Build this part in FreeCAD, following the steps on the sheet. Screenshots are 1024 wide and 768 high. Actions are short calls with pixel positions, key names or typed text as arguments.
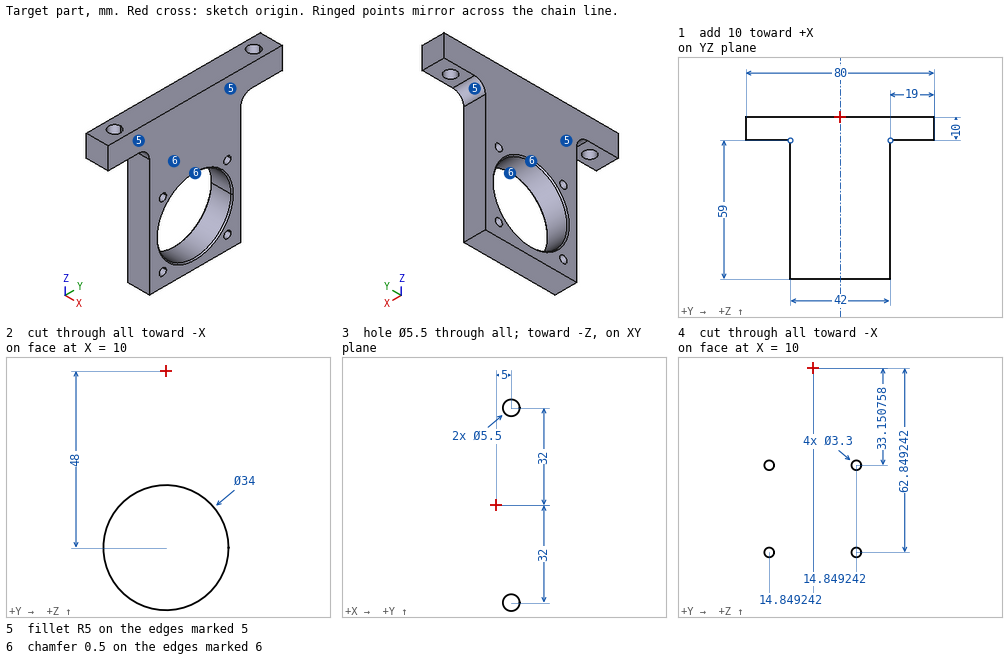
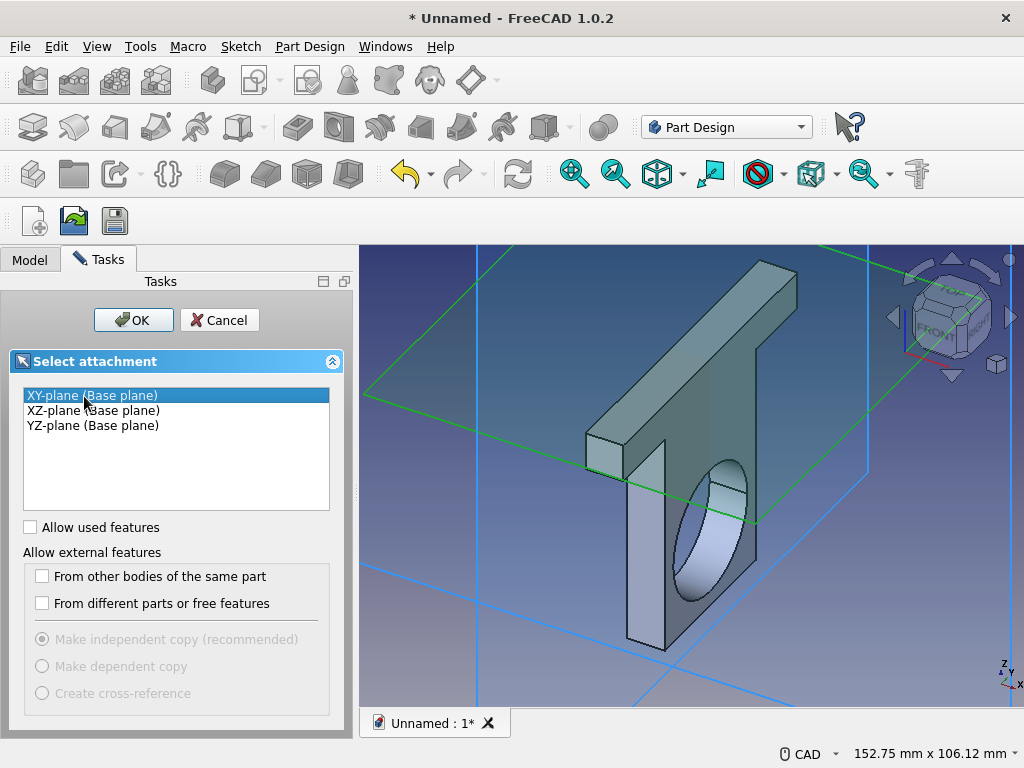
click(134, 320)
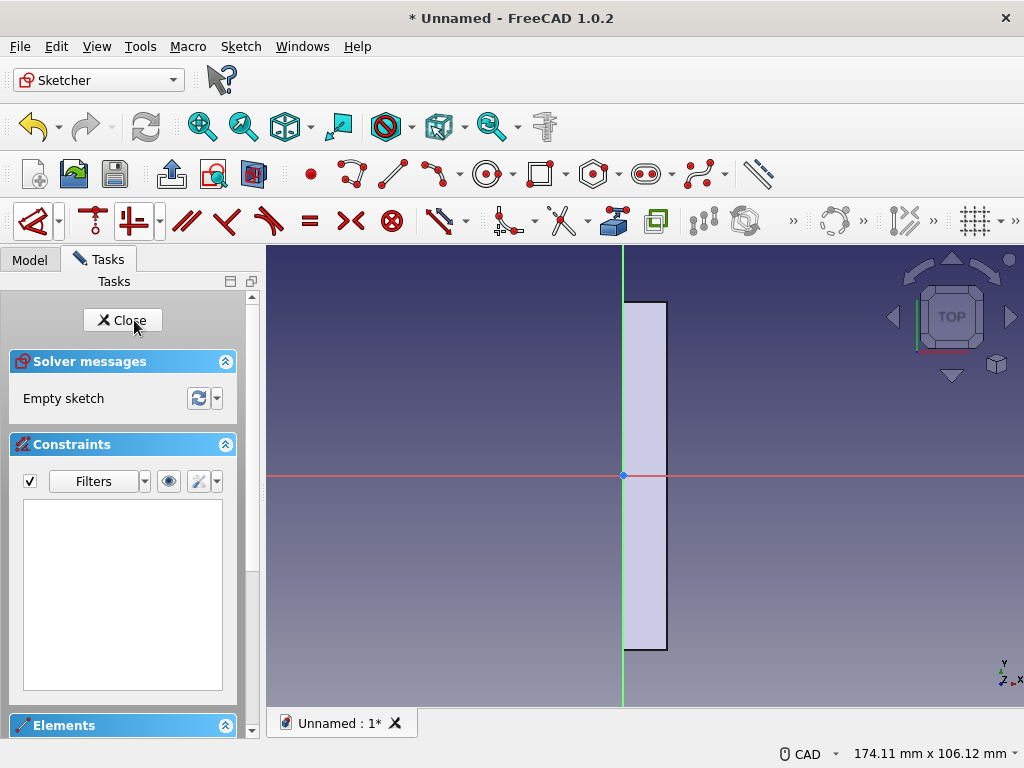
click(486, 174)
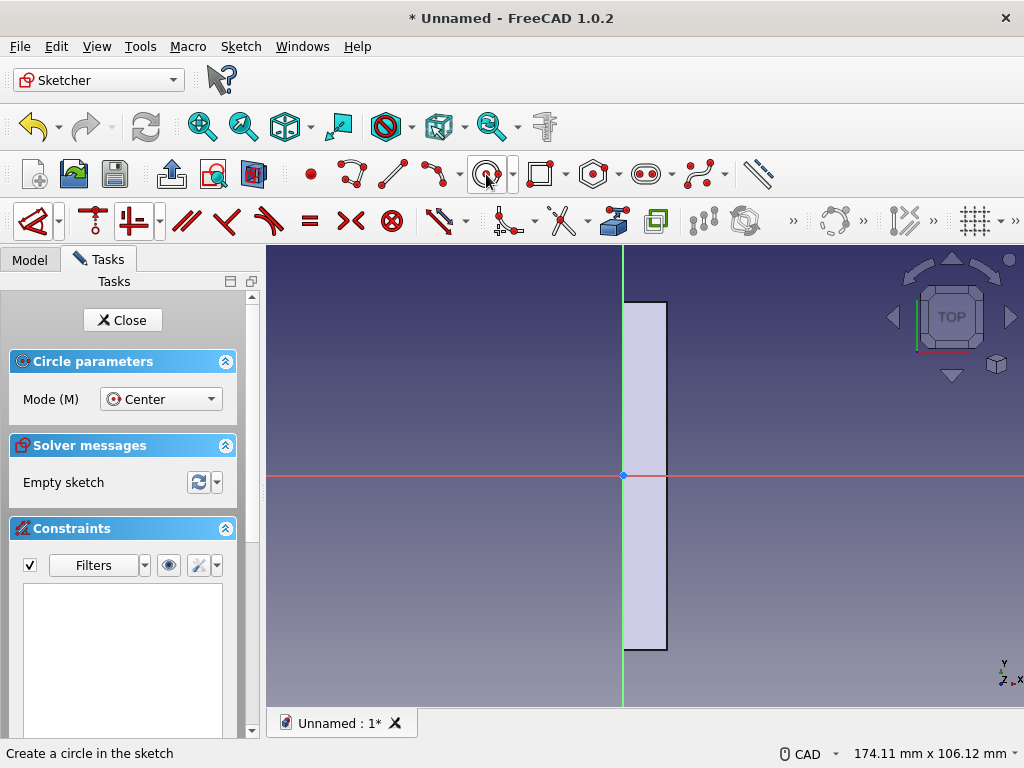
scroll(645, 337, up, 4)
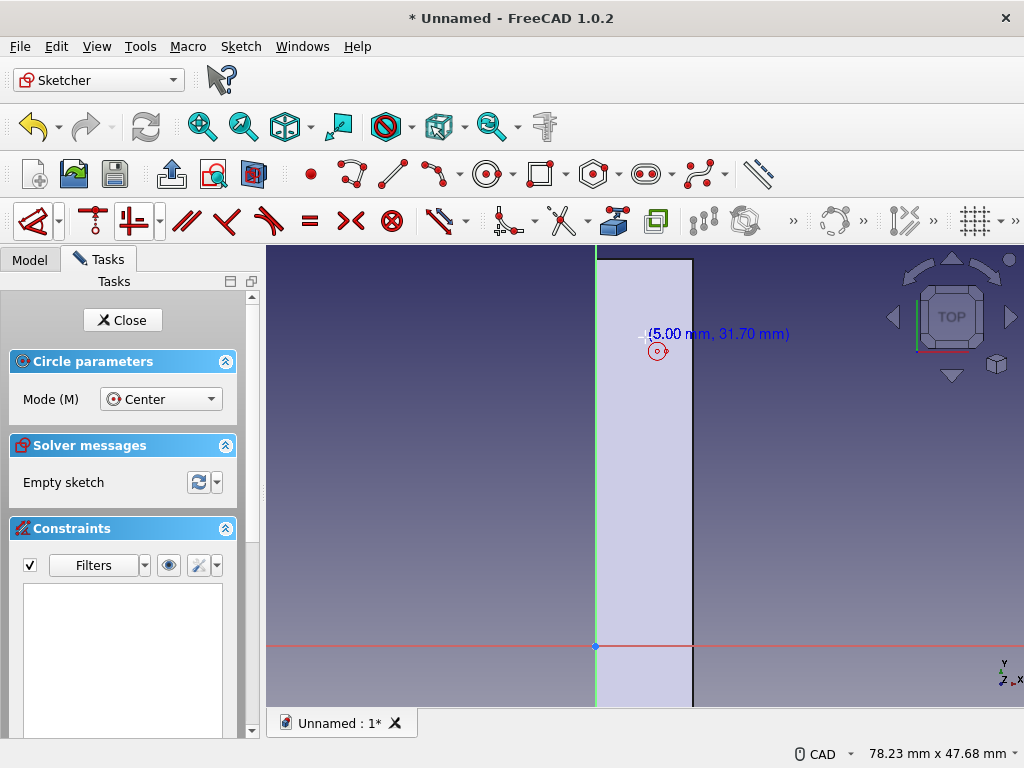
click(644, 336)
move(663, 317)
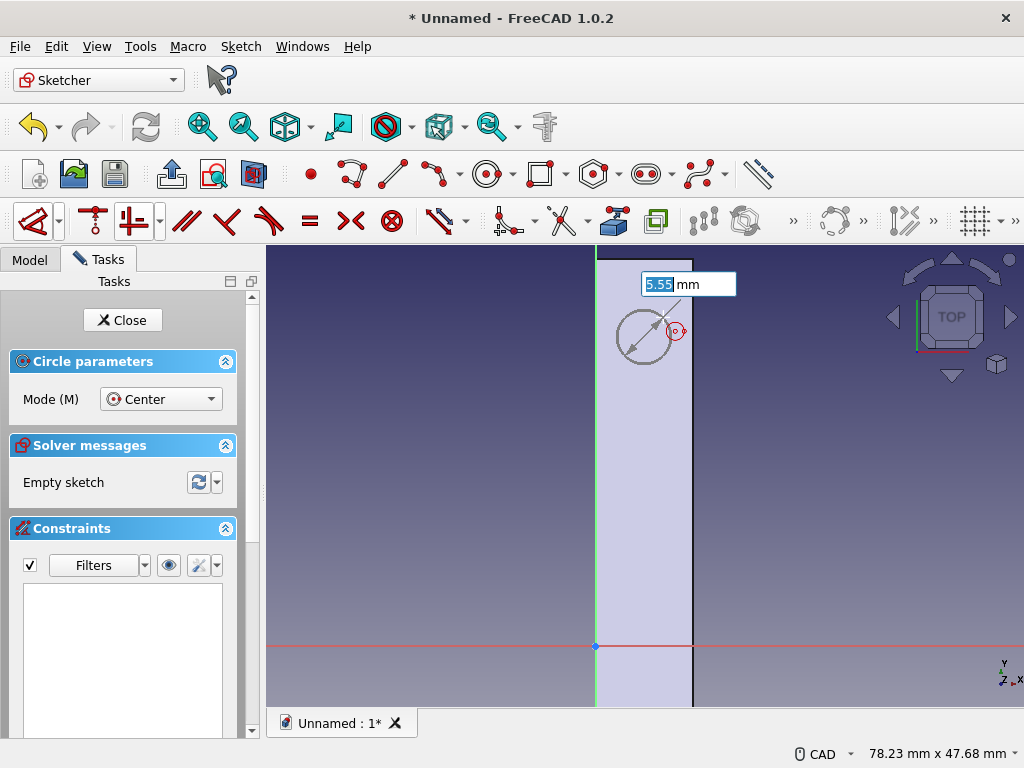
text(5.5)
key(Return)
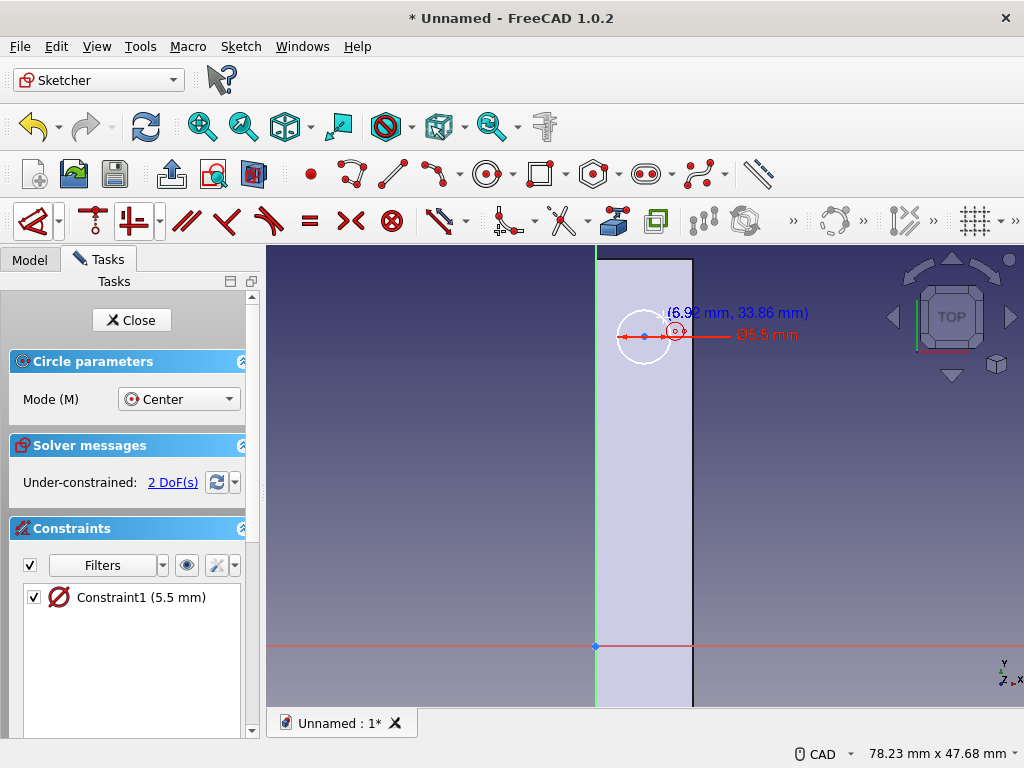
scroll(530, 337, down, 4)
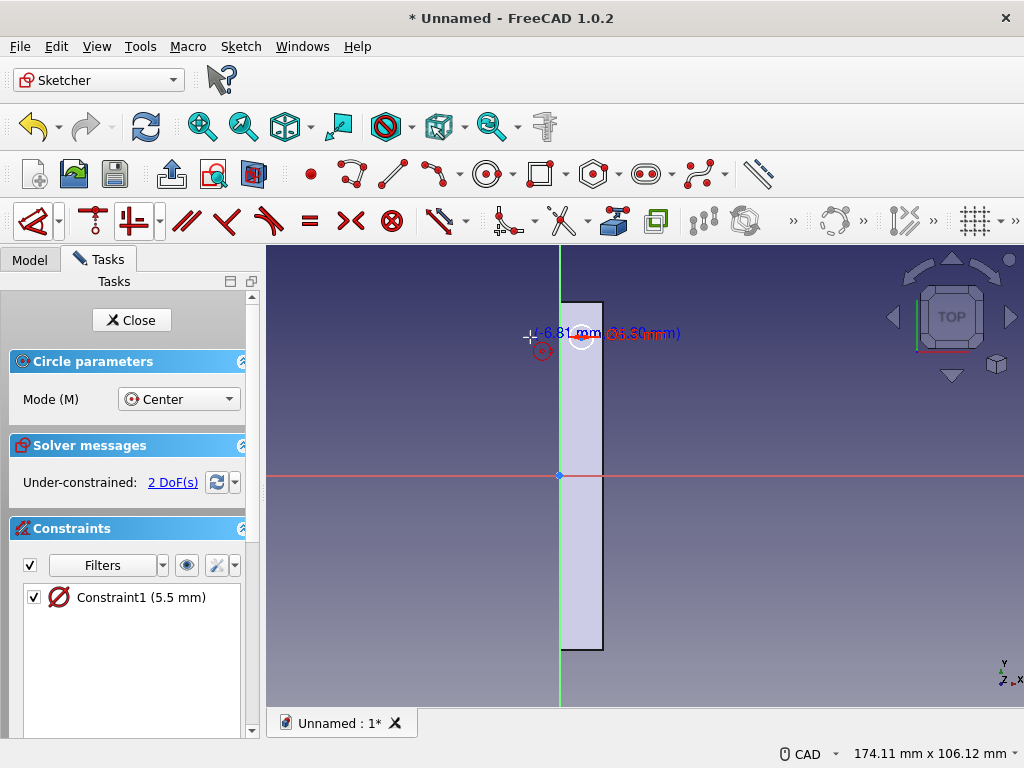
scroll(582, 615, up, 4)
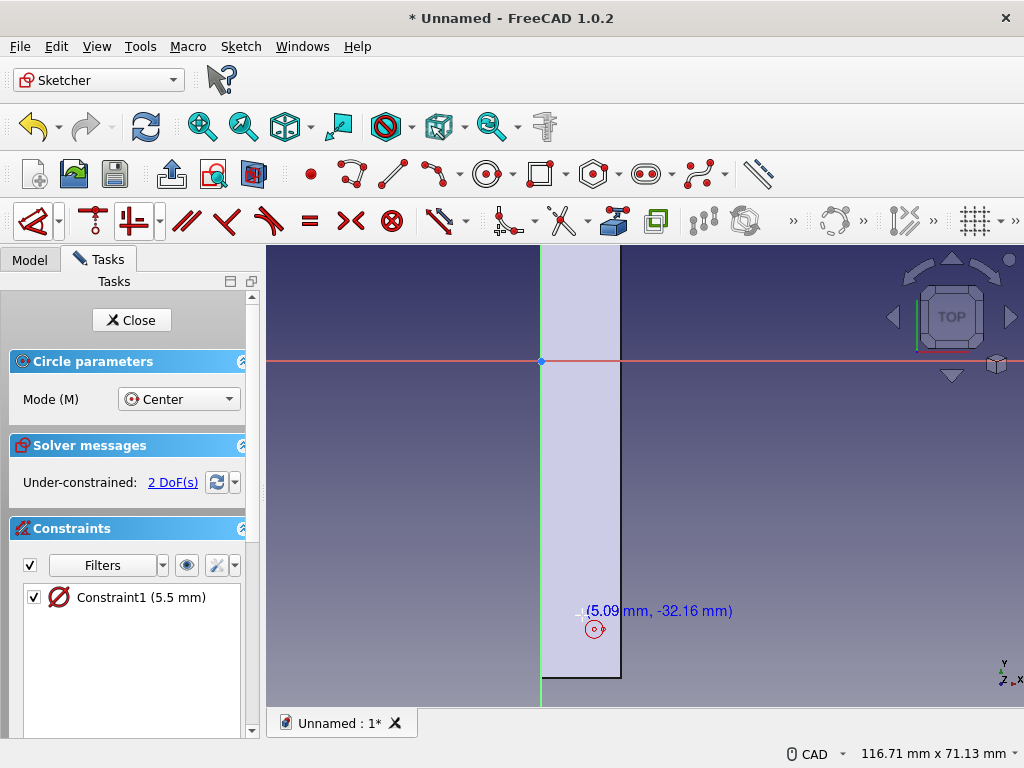
click(581, 615)
move(599, 596)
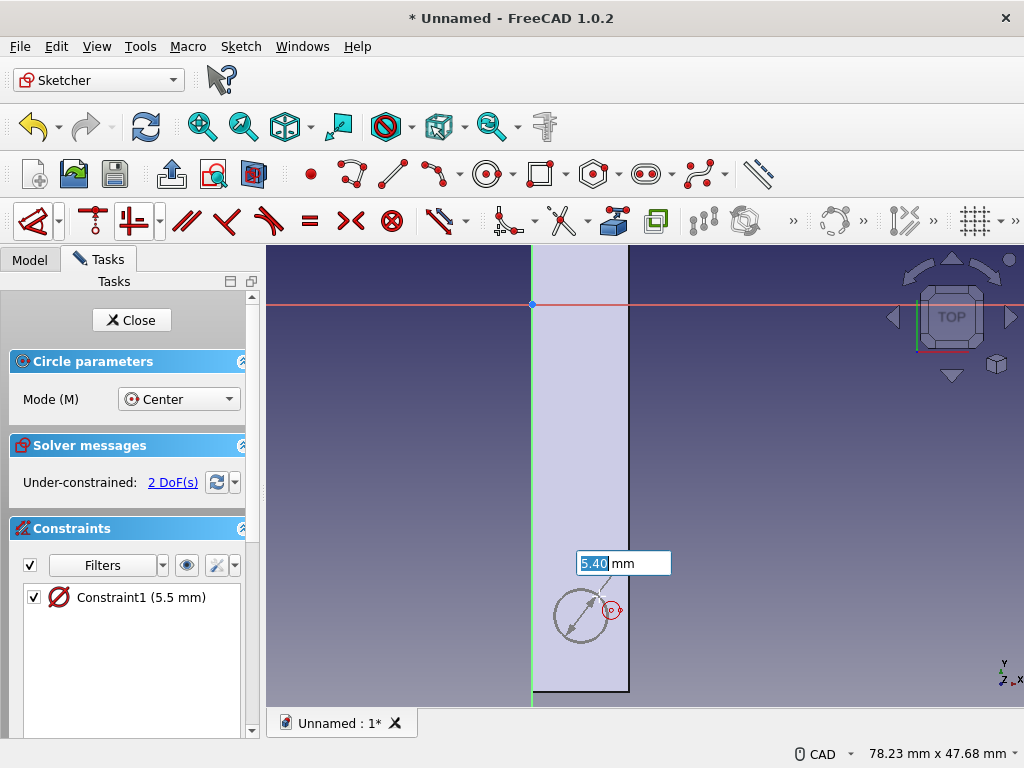
text(5.5)
key(Return)
key(Escape)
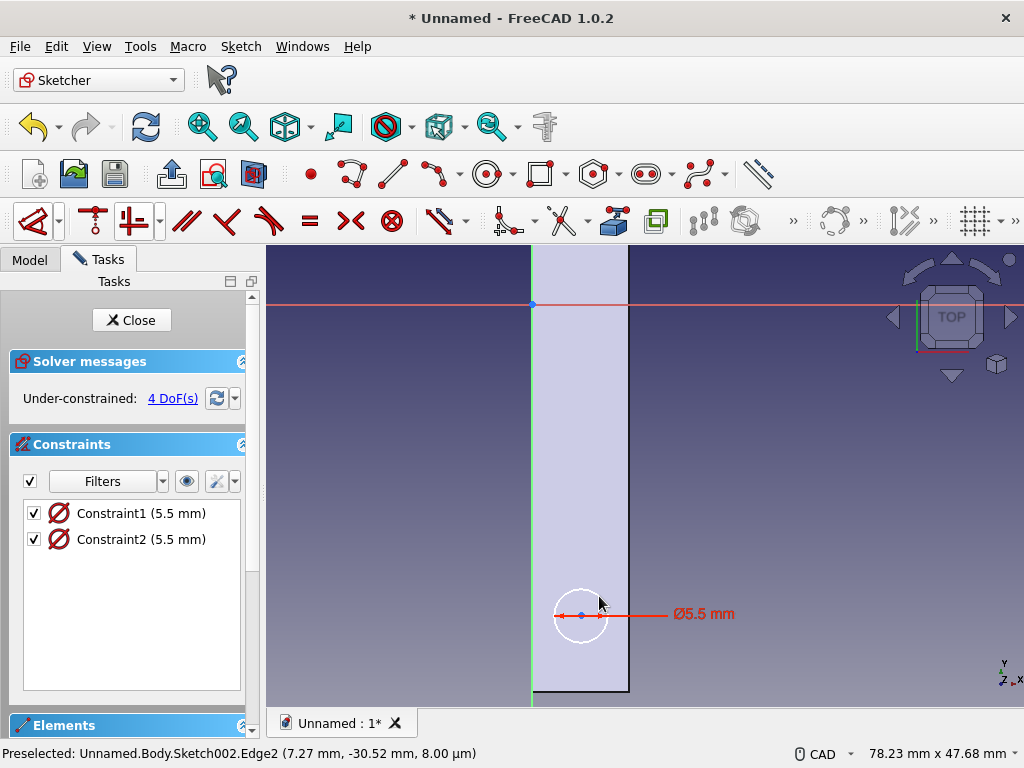
scroll(582, 616, down, 4)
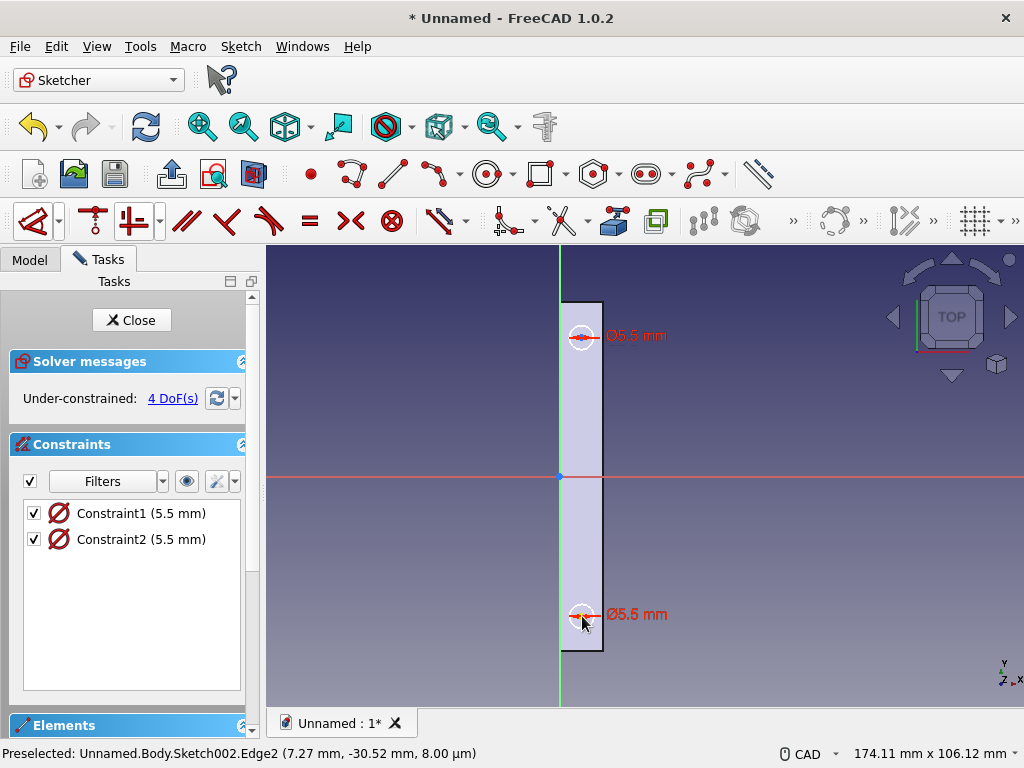
click(581, 338)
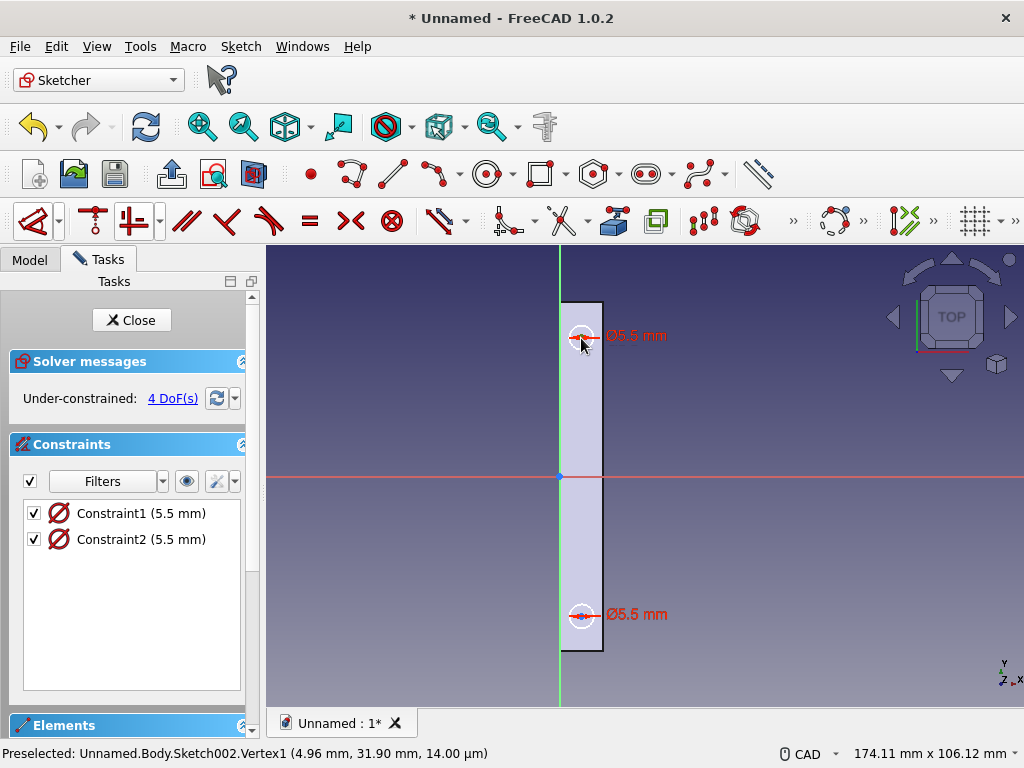
click(582, 616)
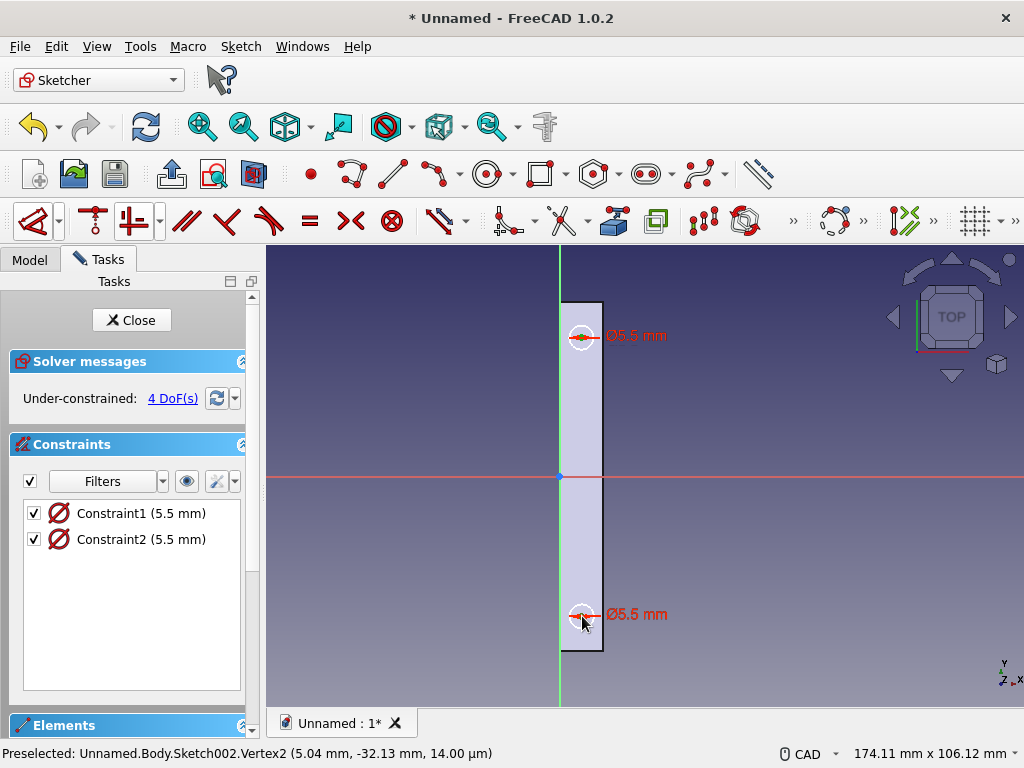
click(160, 222)